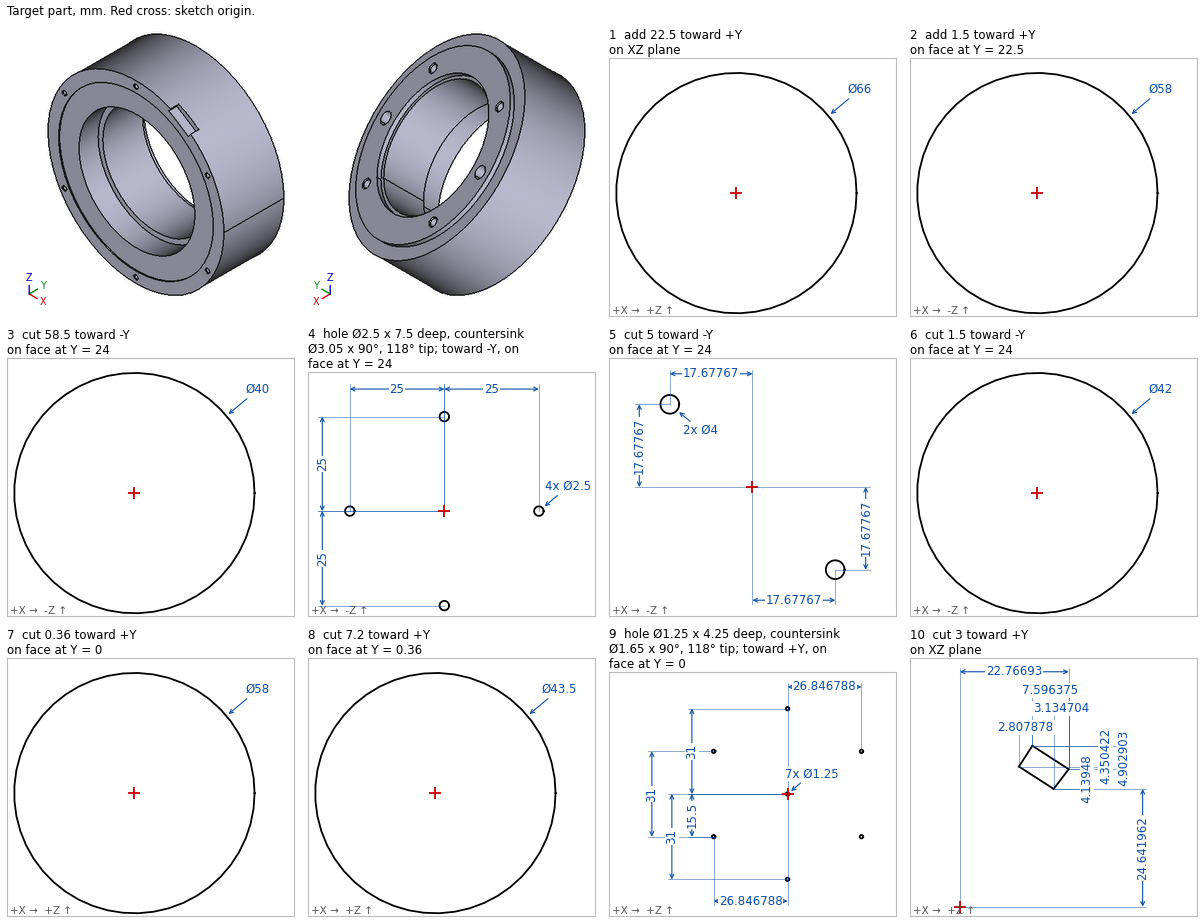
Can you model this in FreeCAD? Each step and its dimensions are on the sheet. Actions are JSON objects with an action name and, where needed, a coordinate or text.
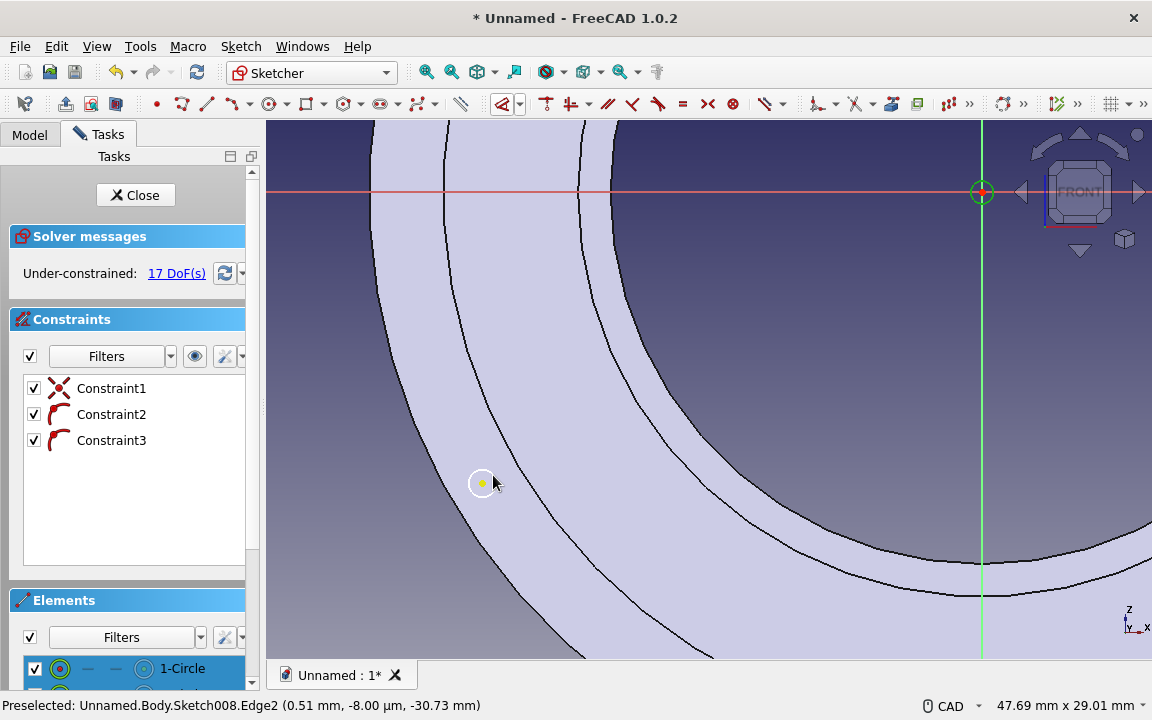
{"action": "left_click", "coordinate": [492, 474]}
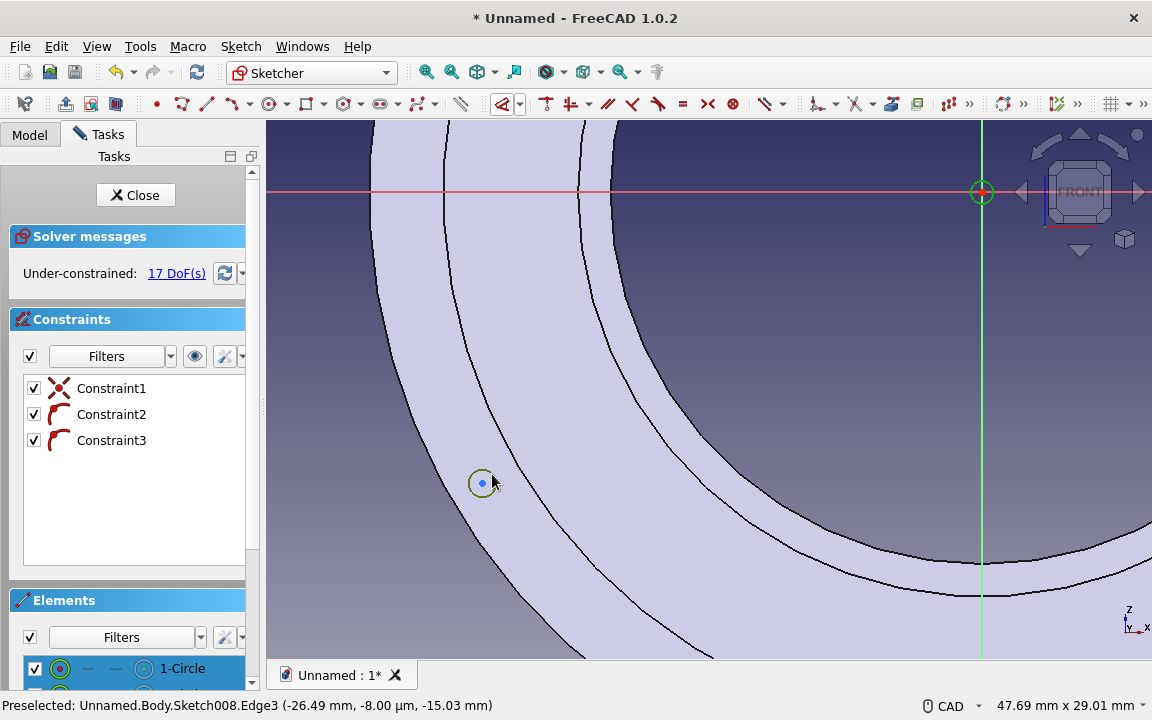
{"action": "scroll", "coordinate": [493, 474], "scroll_direction": "down", "scroll_amount": 6}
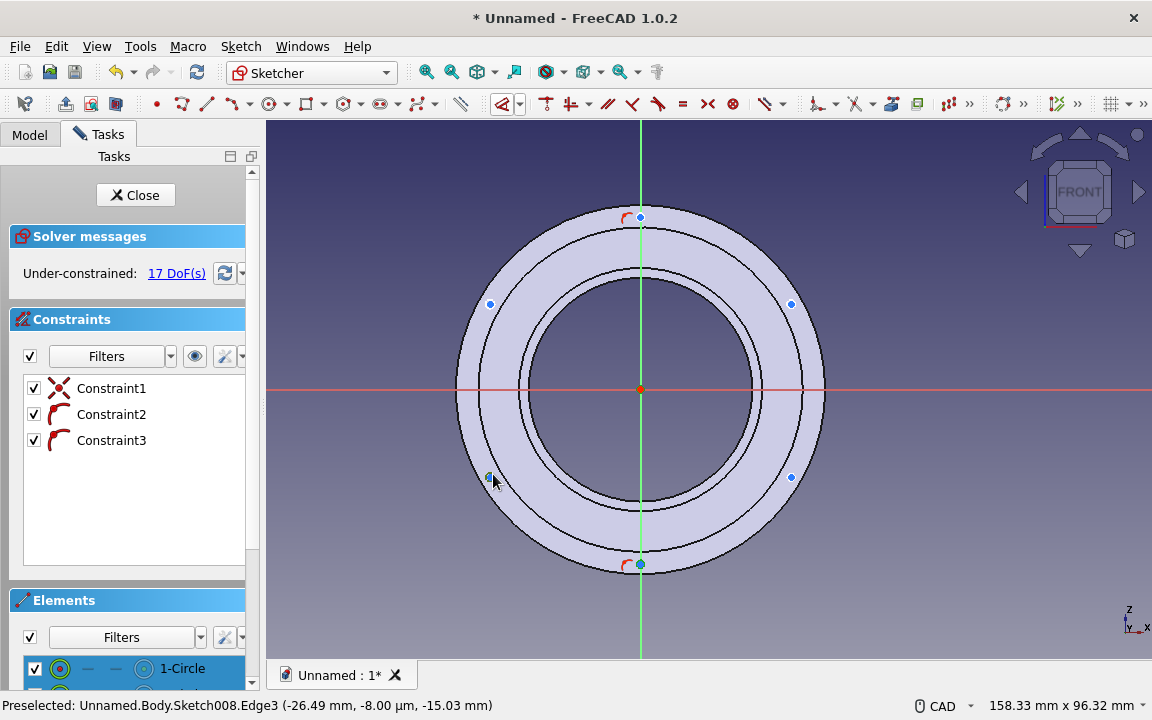
{"action": "scroll", "coordinate": [493, 301], "scroll_direction": "up", "scroll_amount": 6}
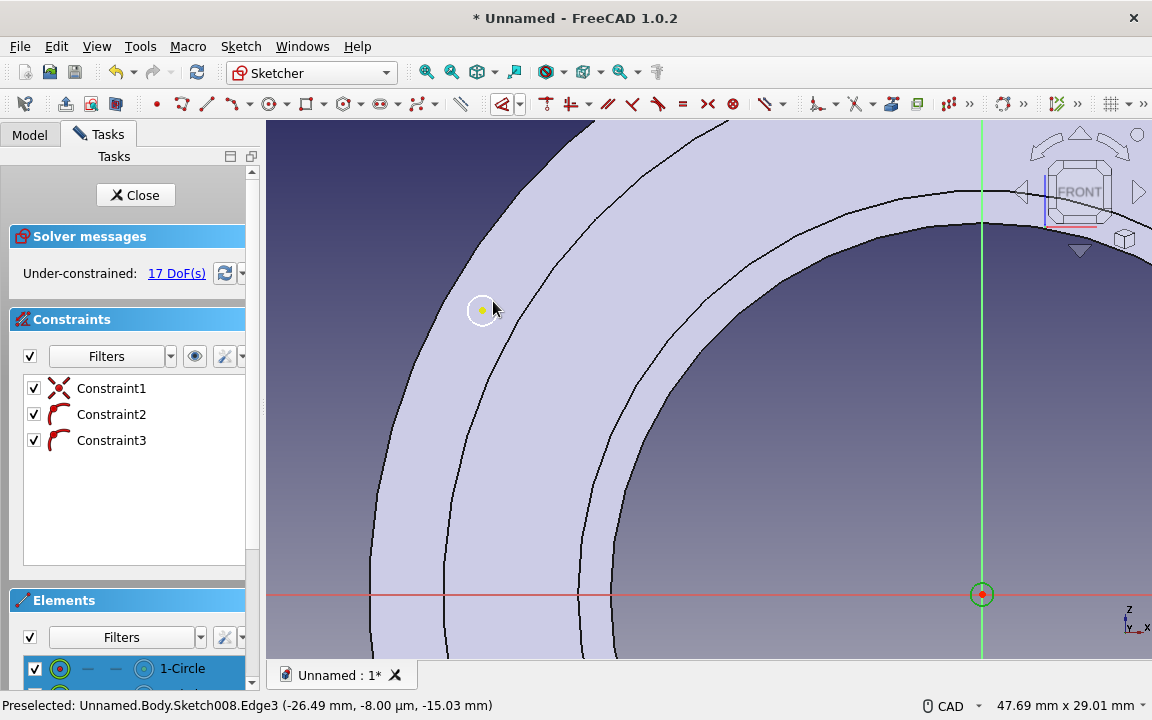
{"action": "left_click", "coordinate": [493, 300]}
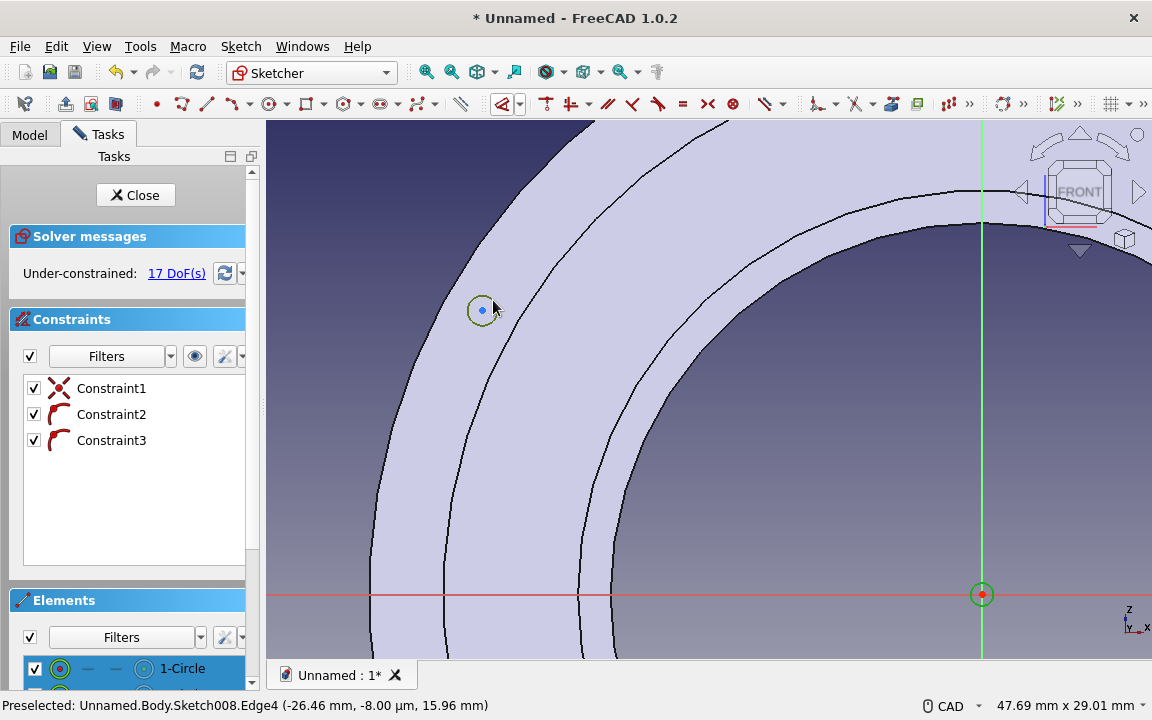
{"action": "scroll", "coordinate": [493, 301], "scroll_direction": "down", "scroll_amount": 6}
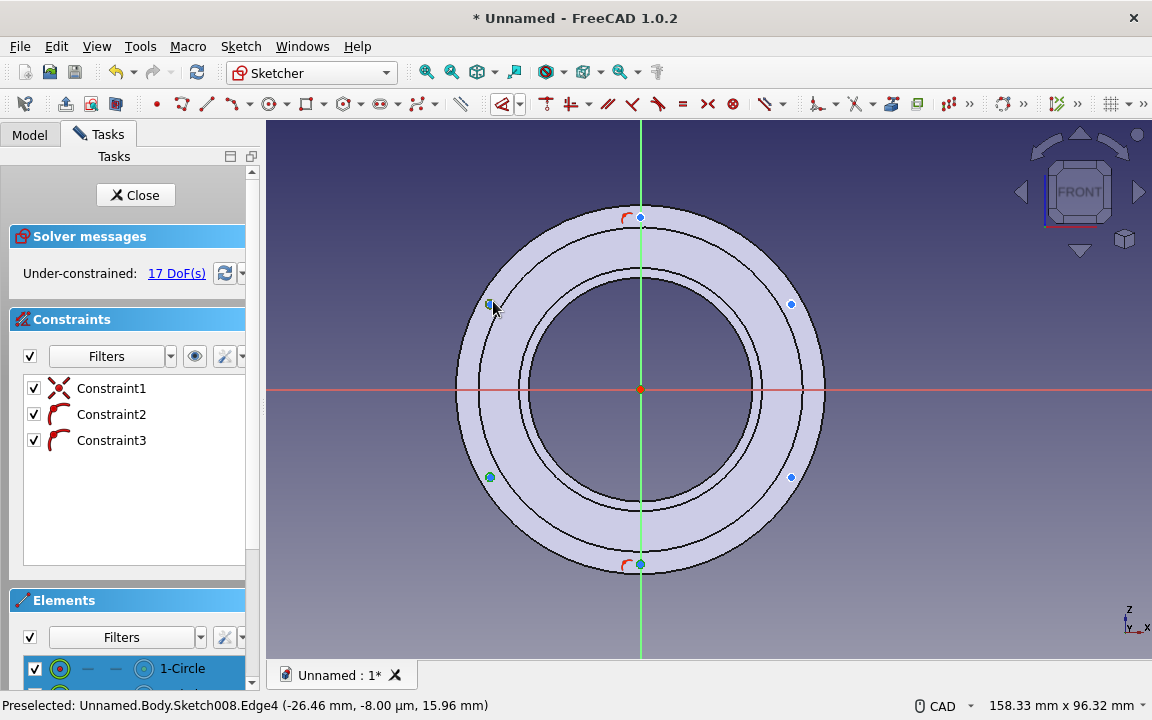
{"action": "scroll", "coordinate": [643, 214], "scroll_direction": "up", "scroll_amount": 9}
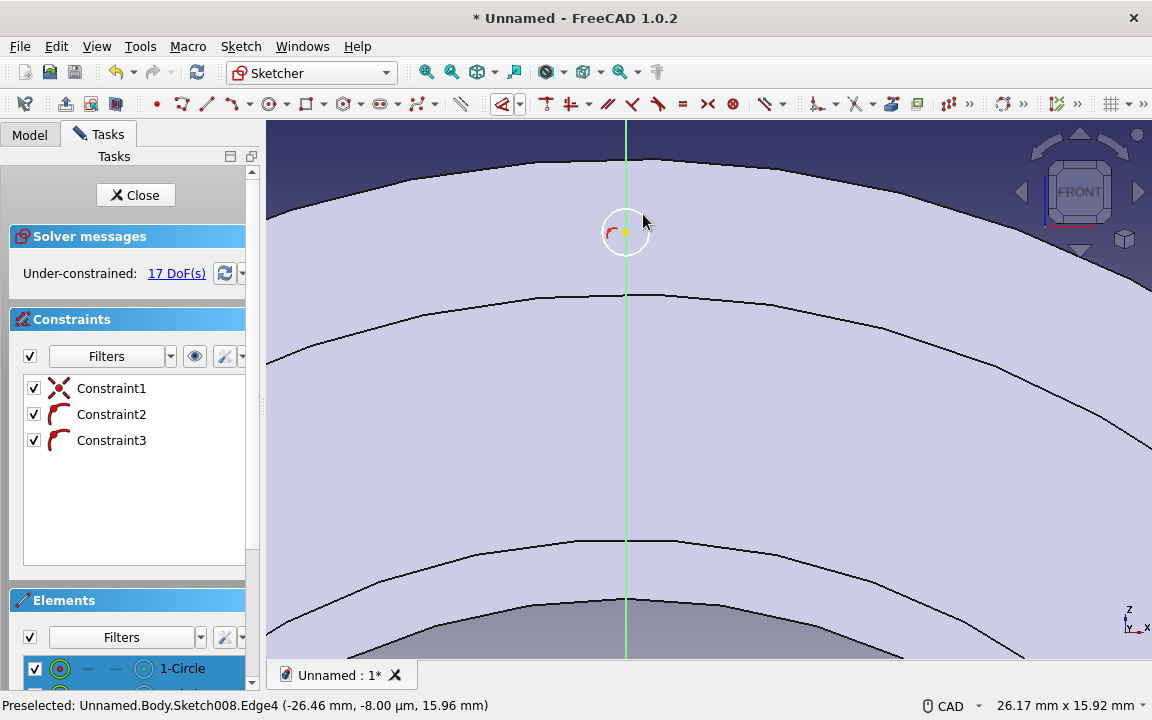
{"action": "left_click", "coordinate": [642, 216]}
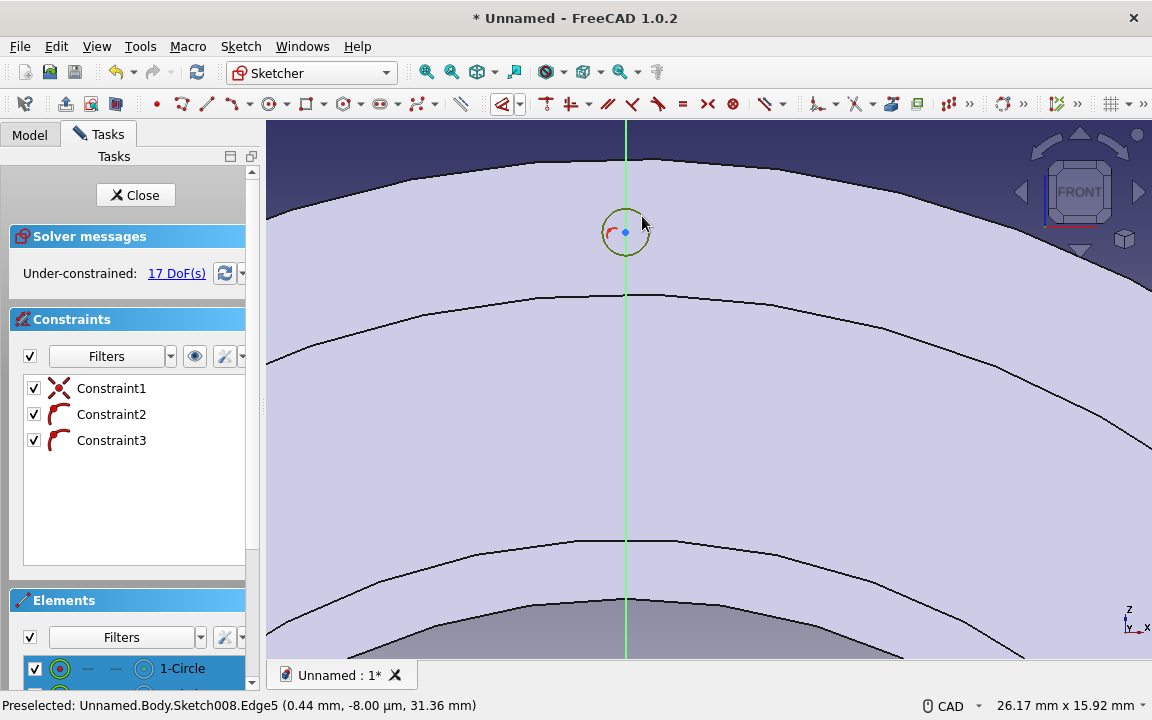
{"action": "scroll", "coordinate": [643, 214], "scroll_direction": "down", "scroll_amount": 9}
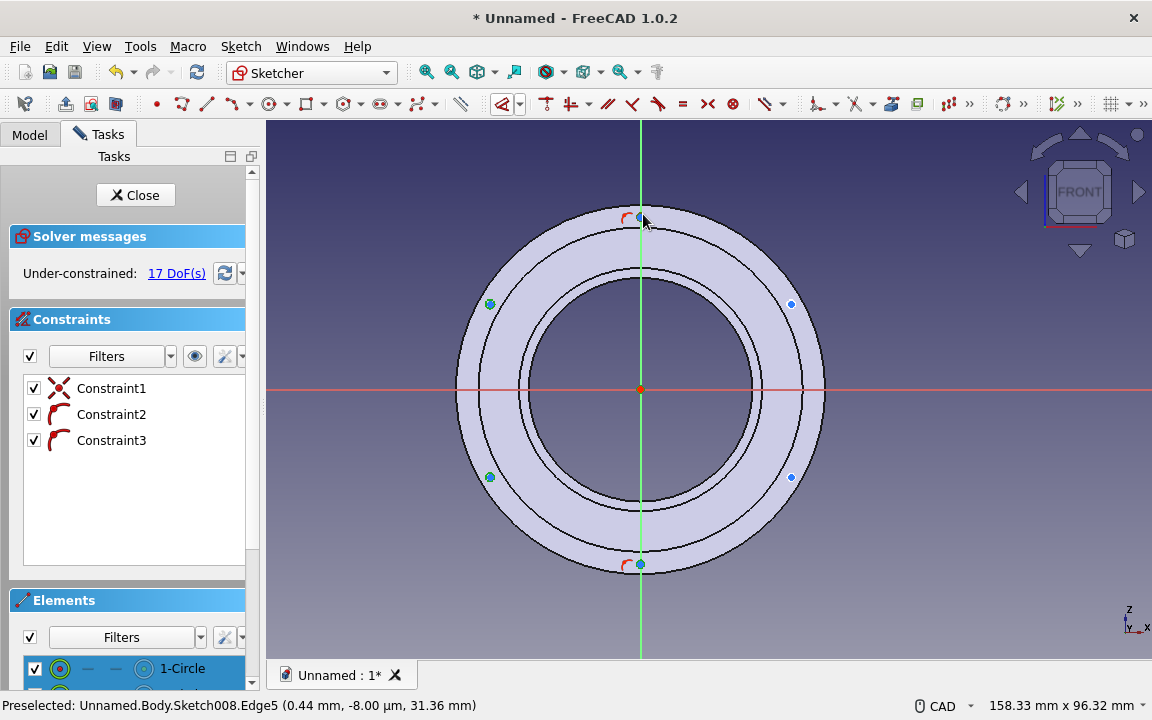
{"action": "scroll", "coordinate": [794, 301], "scroll_direction": "up", "scroll_amount": 7}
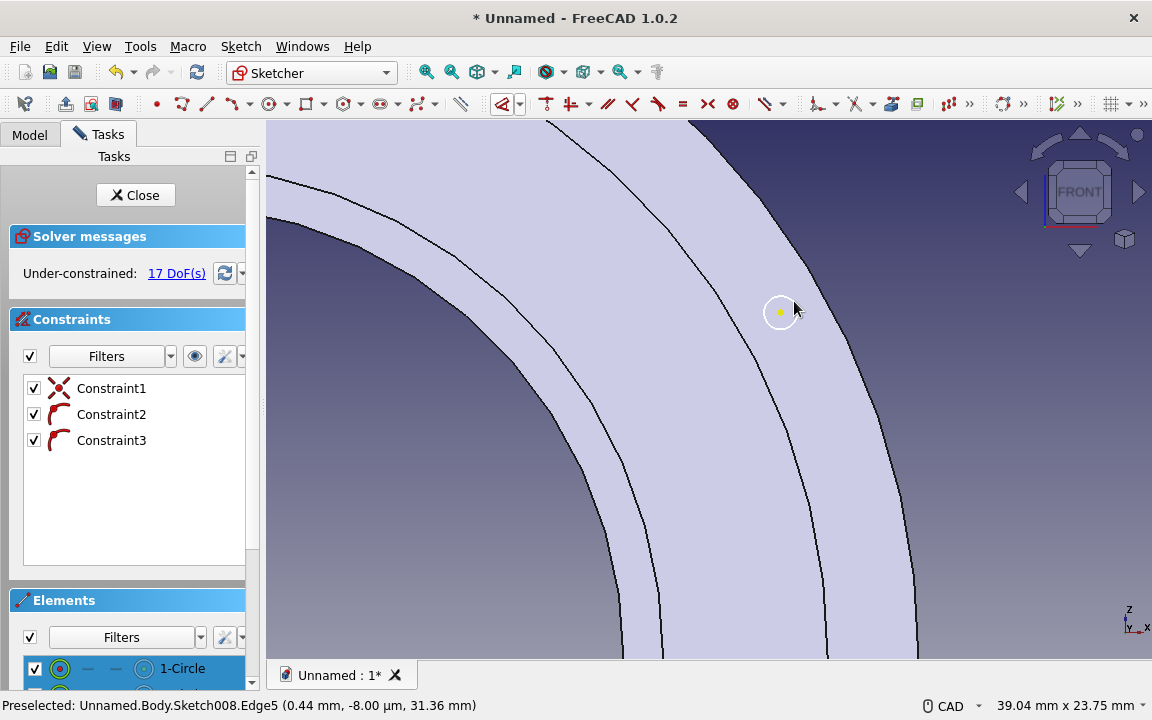
{"action": "left_click", "coordinate": [792, 301]}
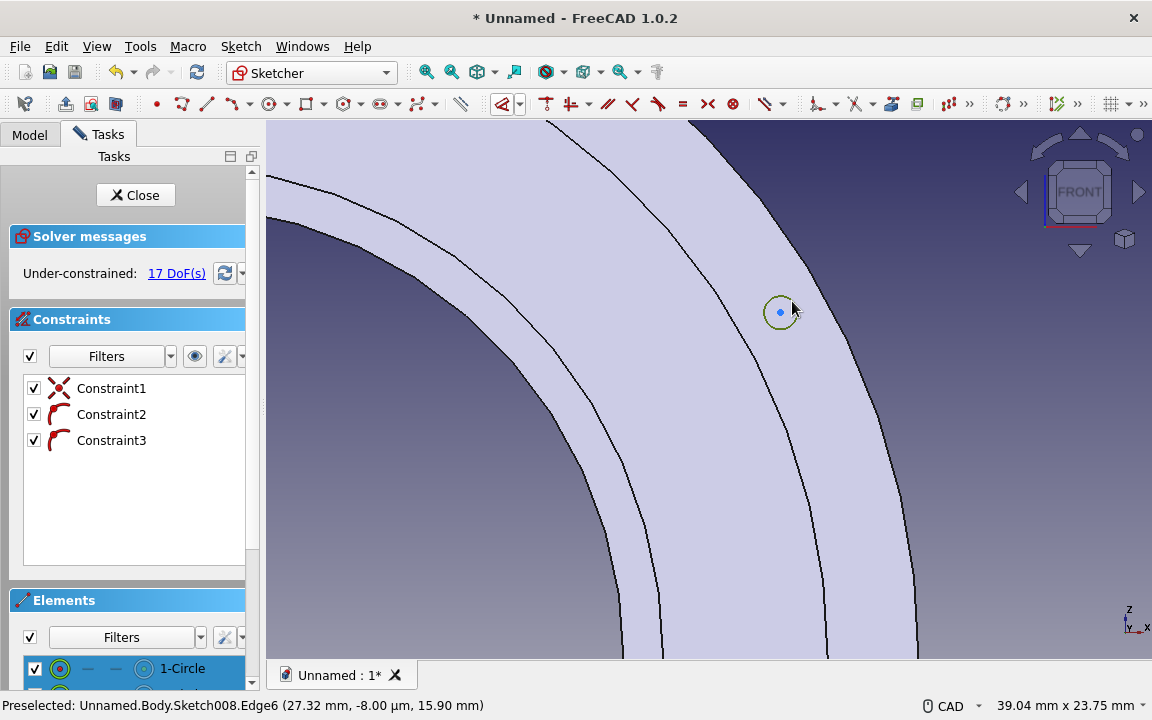
{"action": "scroll", "coordinate": [795, 301], "scroll_direction": "down", "scroll_amount": 7}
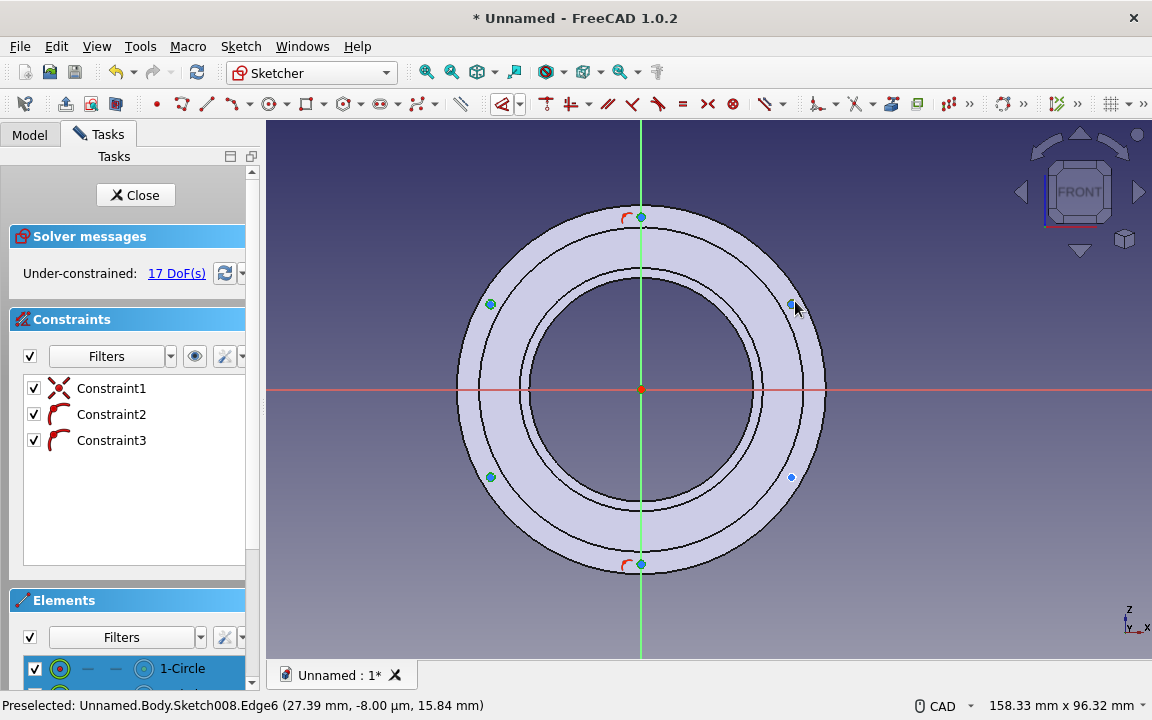
{"action": "scroll", "coordinate": [795, 475], "scroll_direction": "up", "scroll_amount": 7}